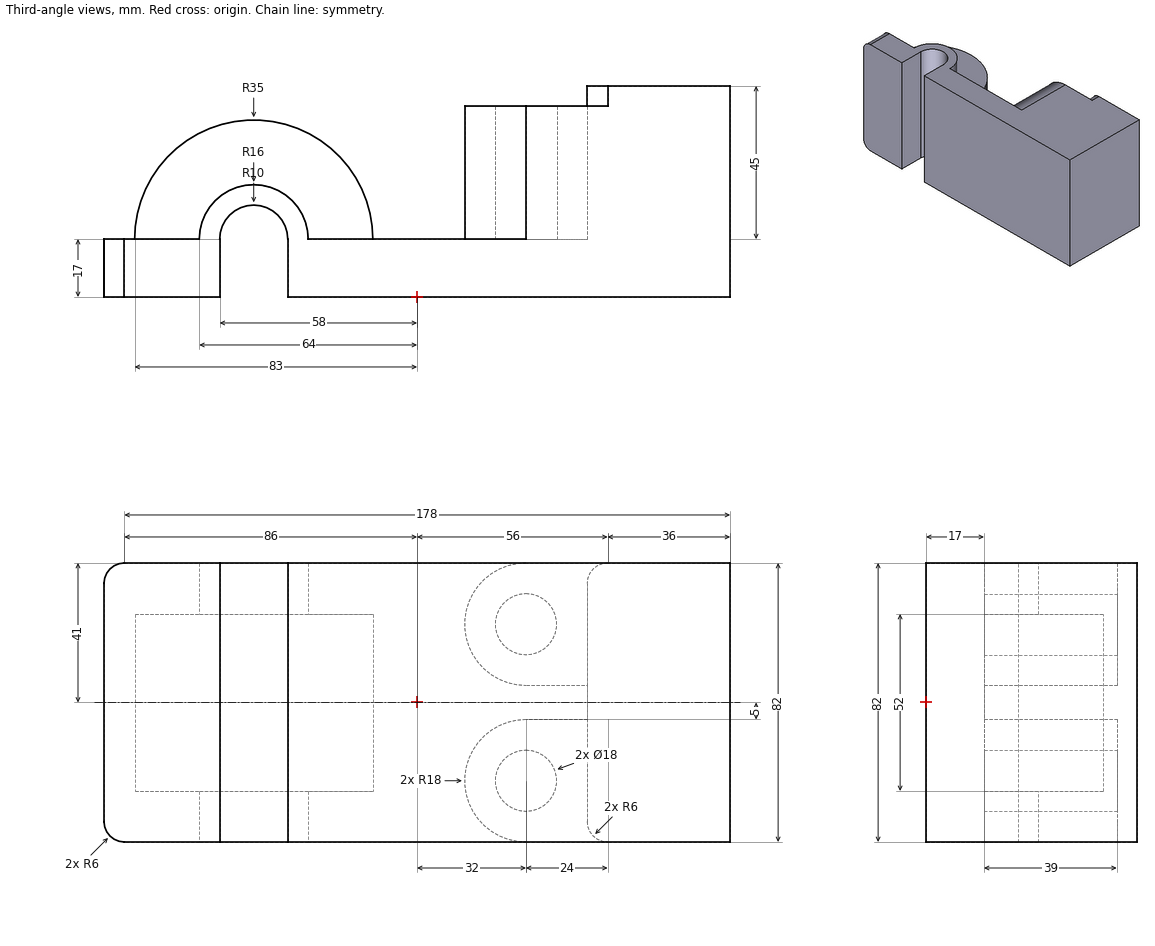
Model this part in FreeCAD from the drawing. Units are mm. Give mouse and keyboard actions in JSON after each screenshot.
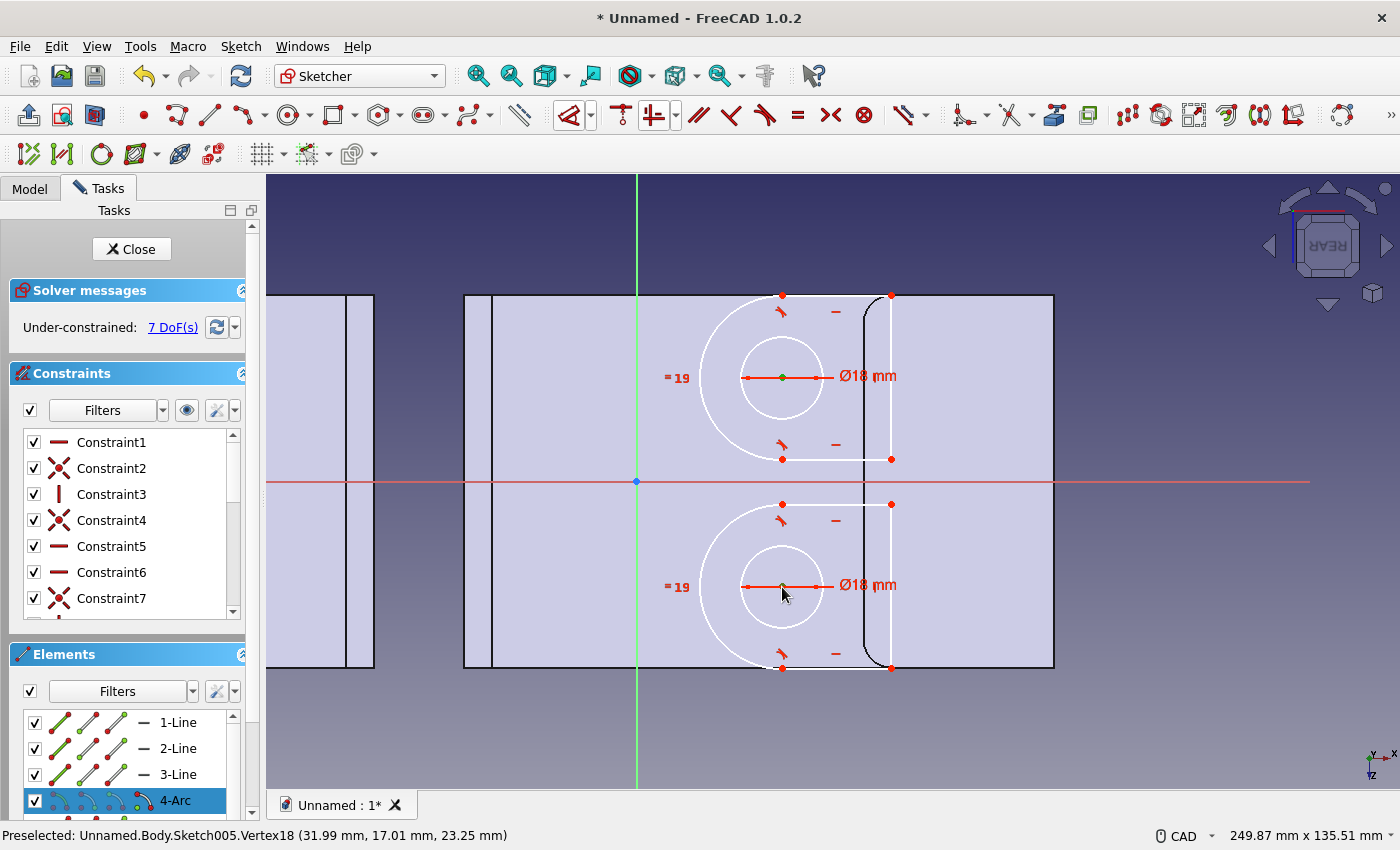
{"action": "left_click", "coordinate": [361, 481]}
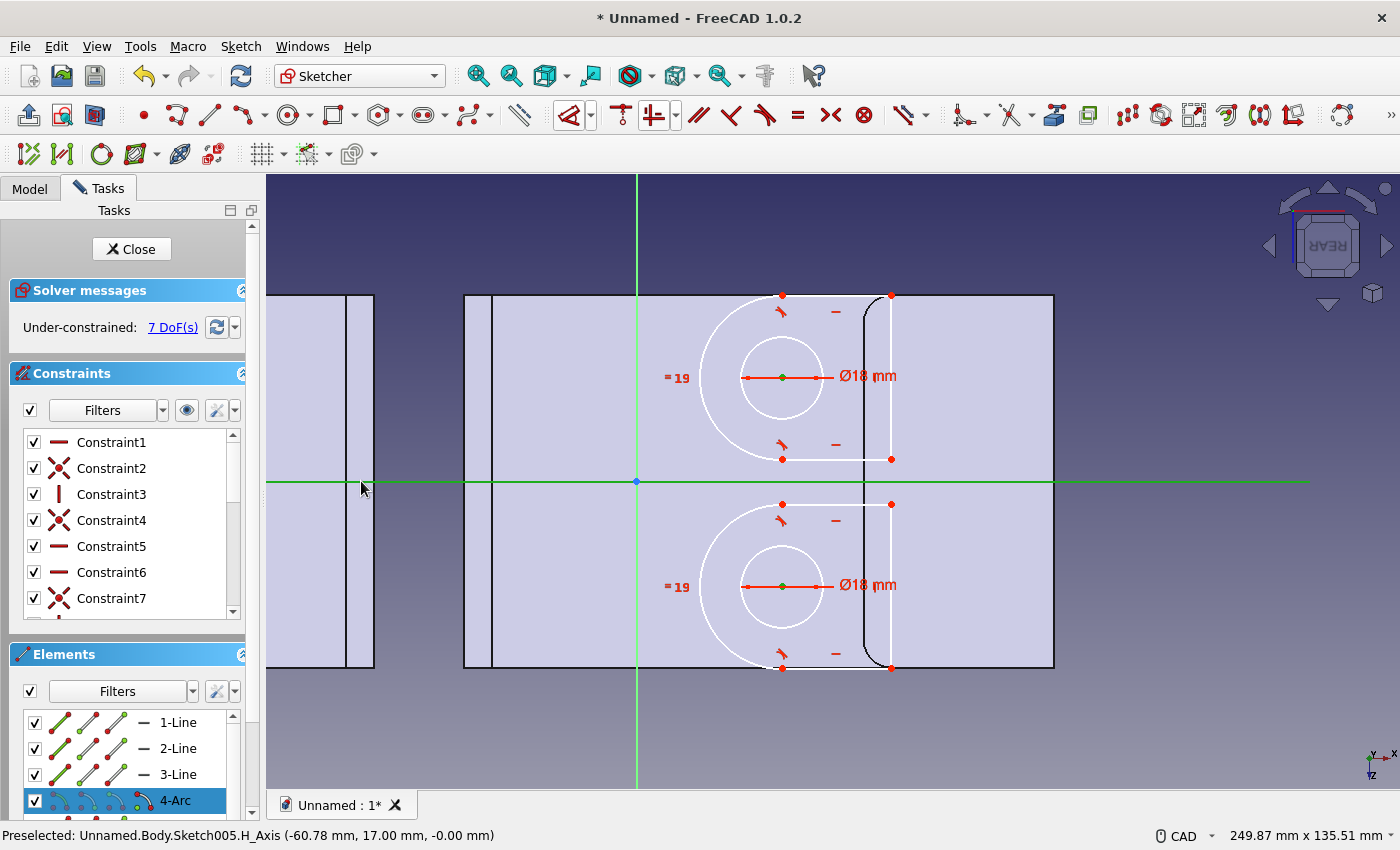
{"action": "left_click", "coordinate": [831, 116]}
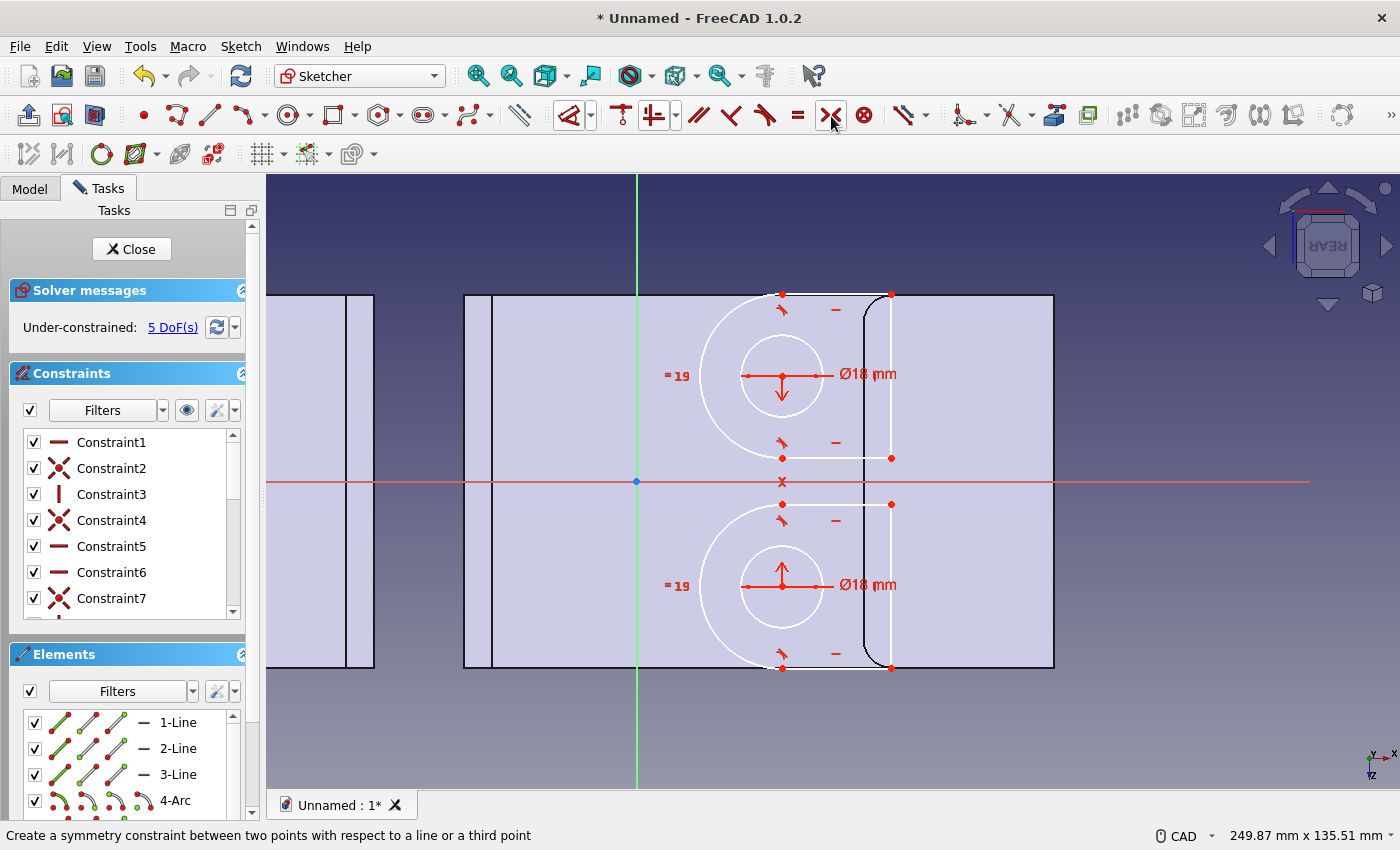
{"action": "left_click", "coordinate": [716, 328]}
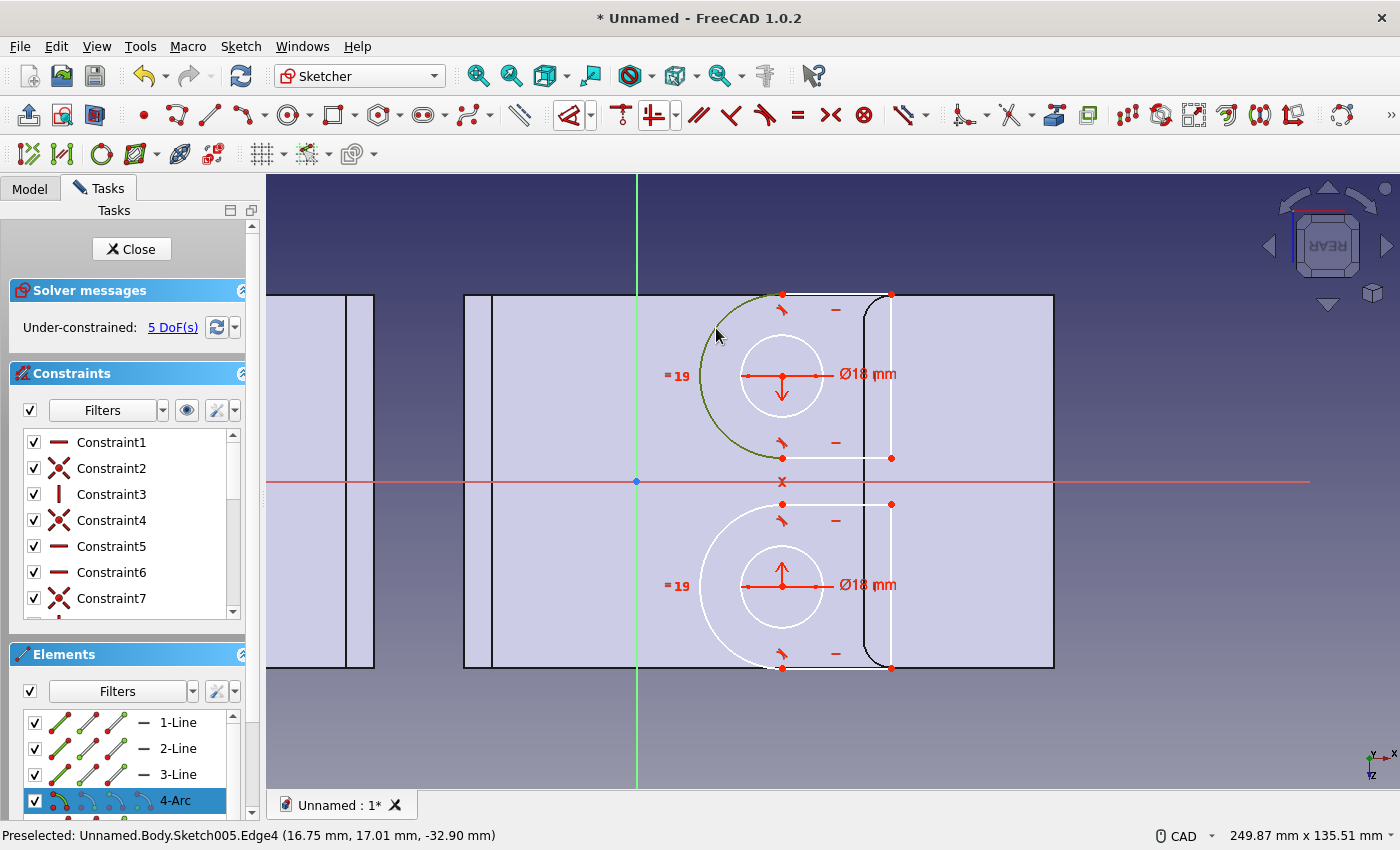
{"action": "key", "text": "k r"}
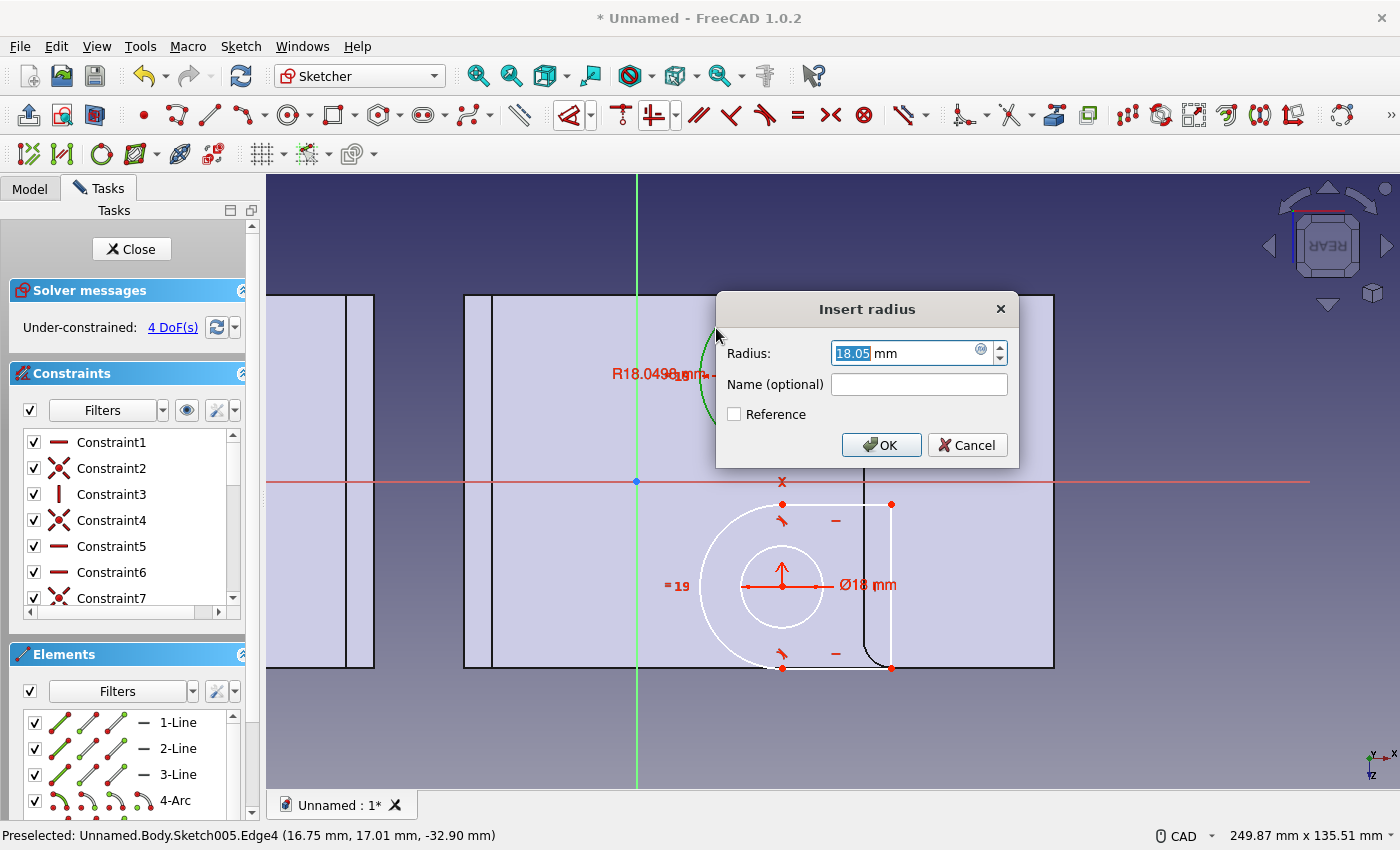
{"action": "type", "text": "18"}
{"action": "key", "text": "Return"}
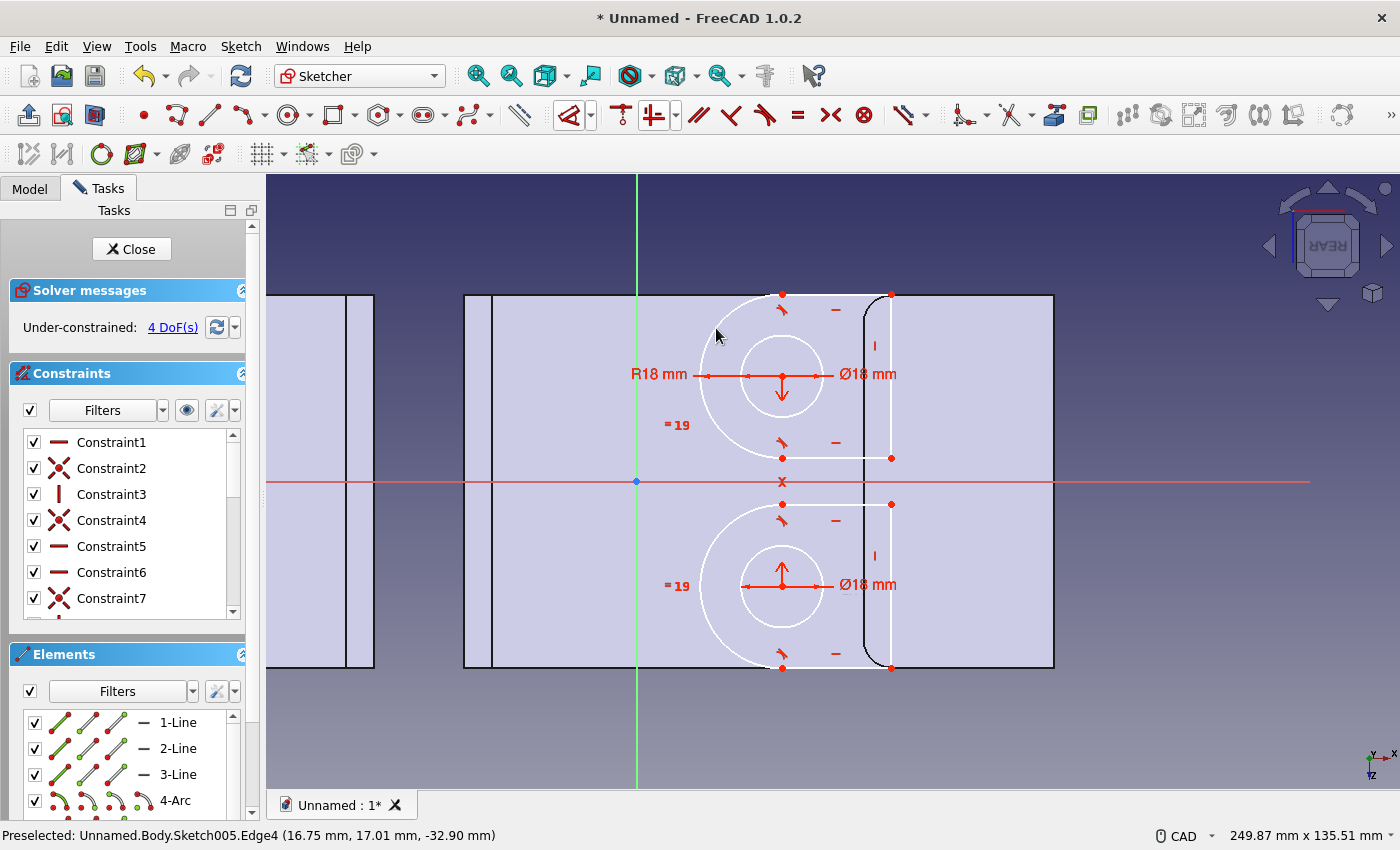
{"action": "left_click", "coordinate": [815, 458]}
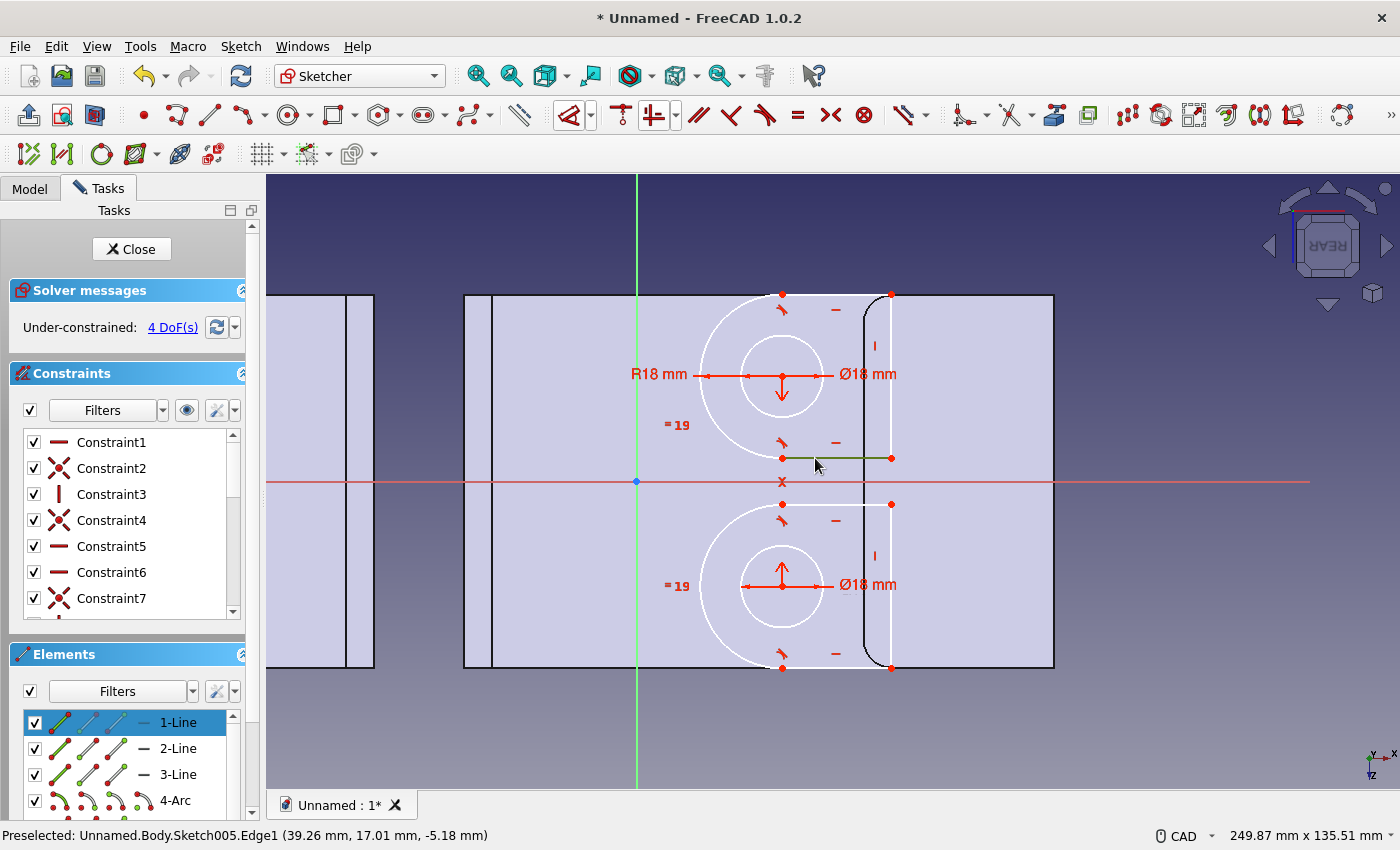
{"action": "left_click", "coordinate": [590, 116]}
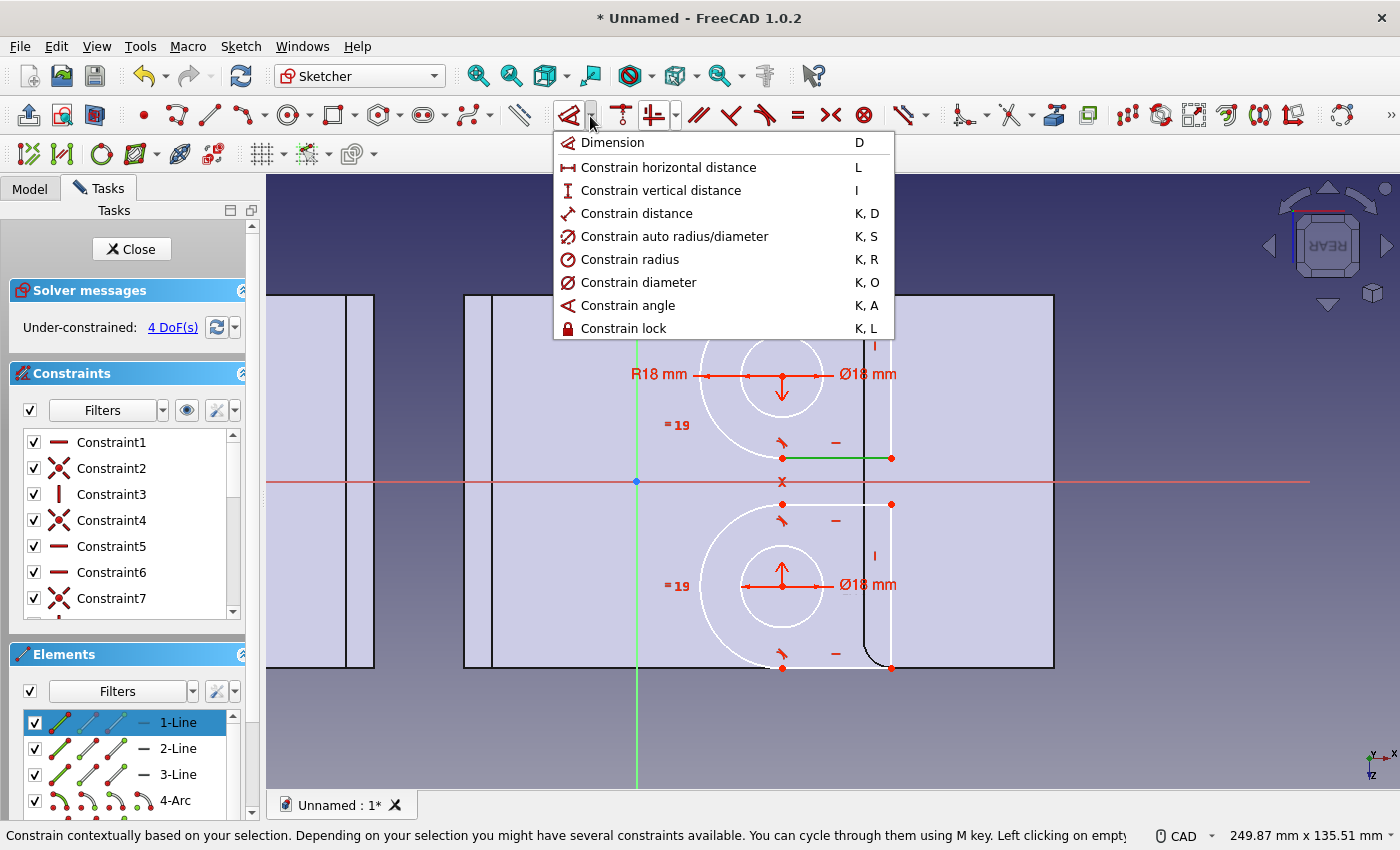
{"action": "left_click", "coordinate": [724, 168]}